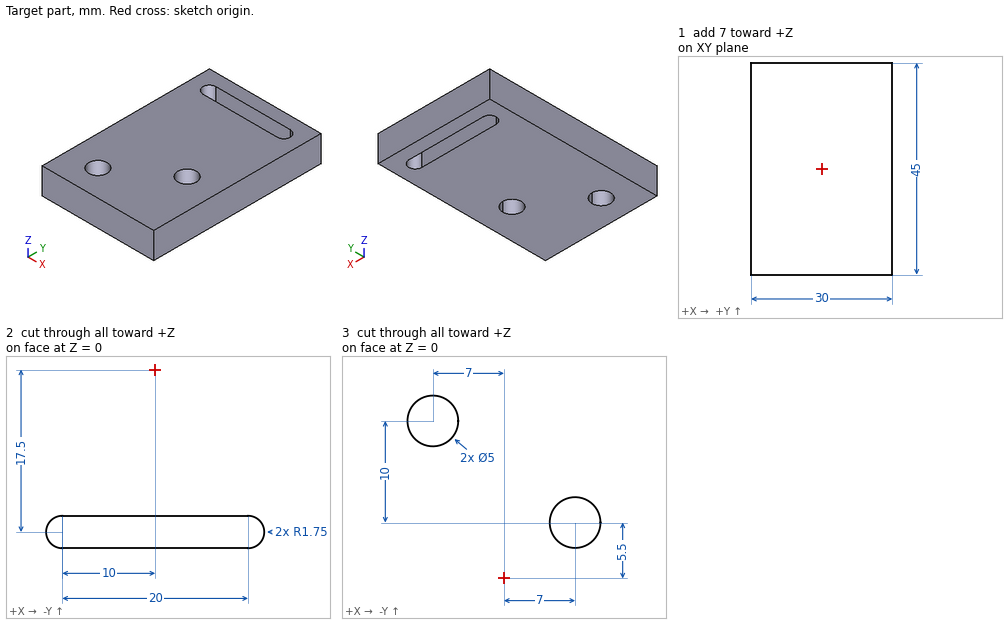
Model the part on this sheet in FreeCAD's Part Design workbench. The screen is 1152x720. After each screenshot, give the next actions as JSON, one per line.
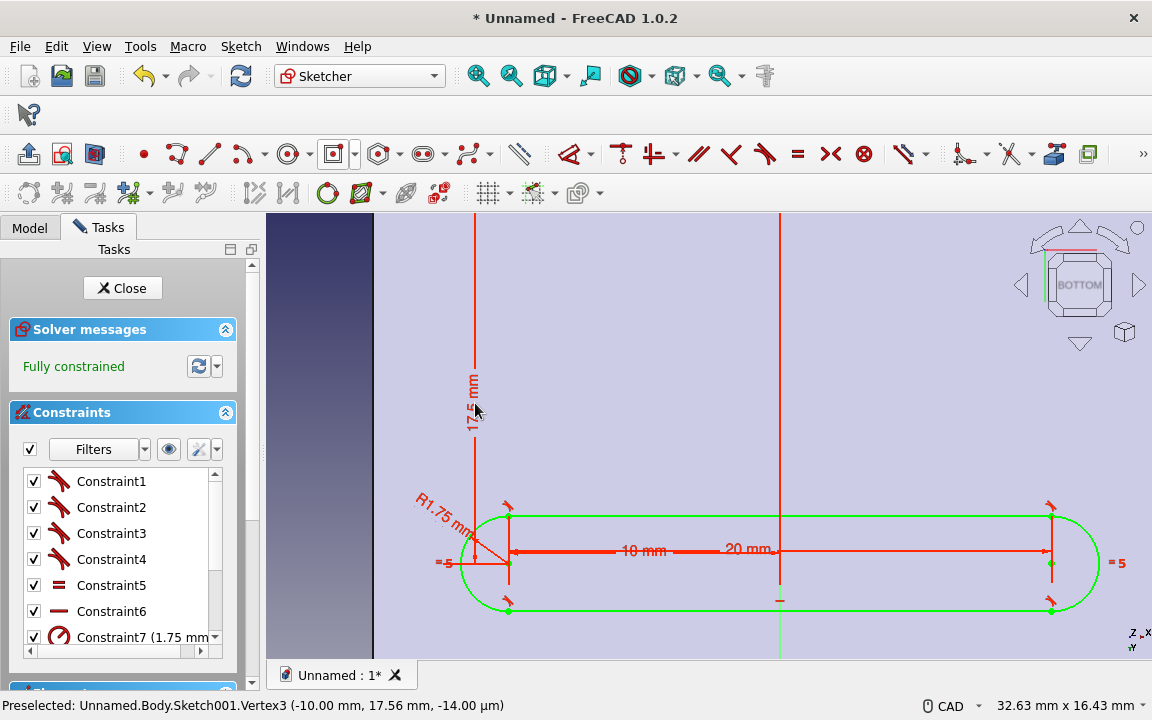
{"action": "left_click", "coordinate": [123, 288]}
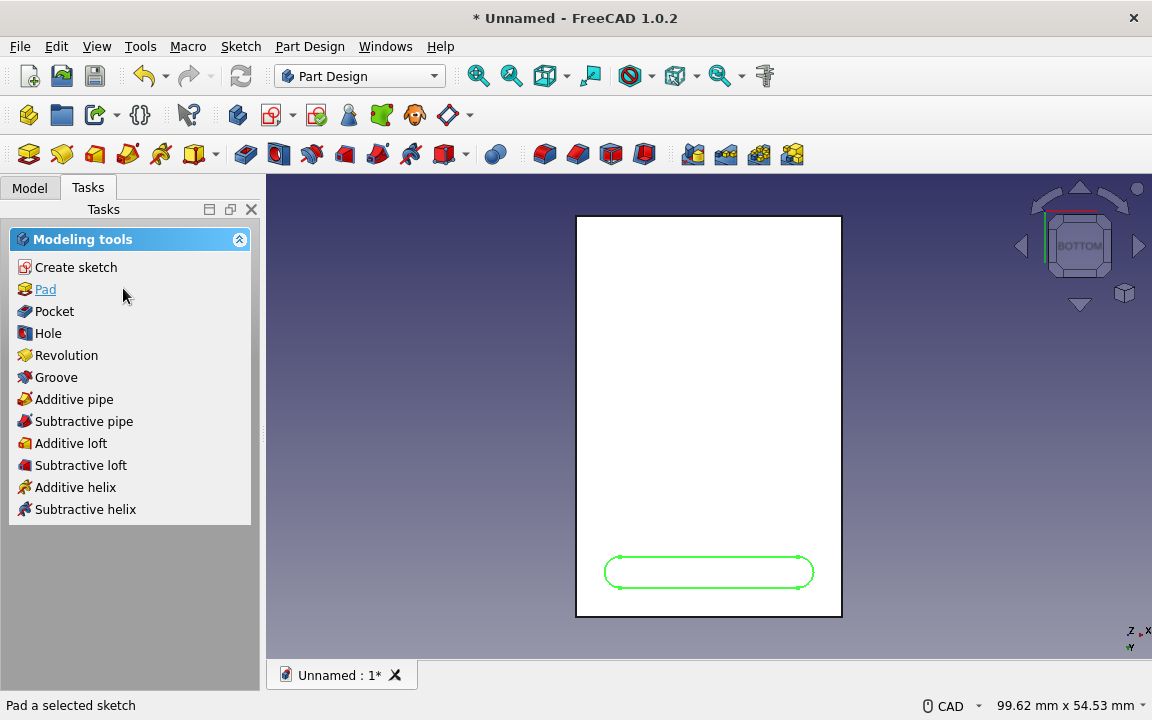
{"action": "left_click", "coordinate": [246, 154]}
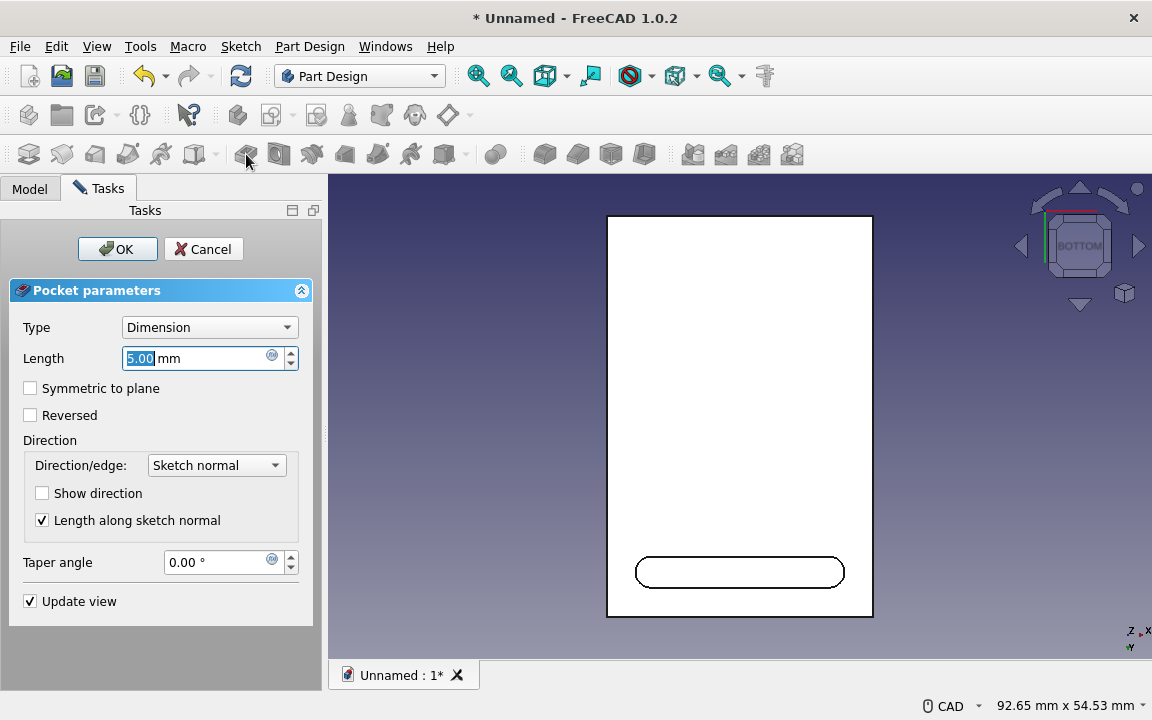
{"action": "left_click", "coordinate": [210, 328]}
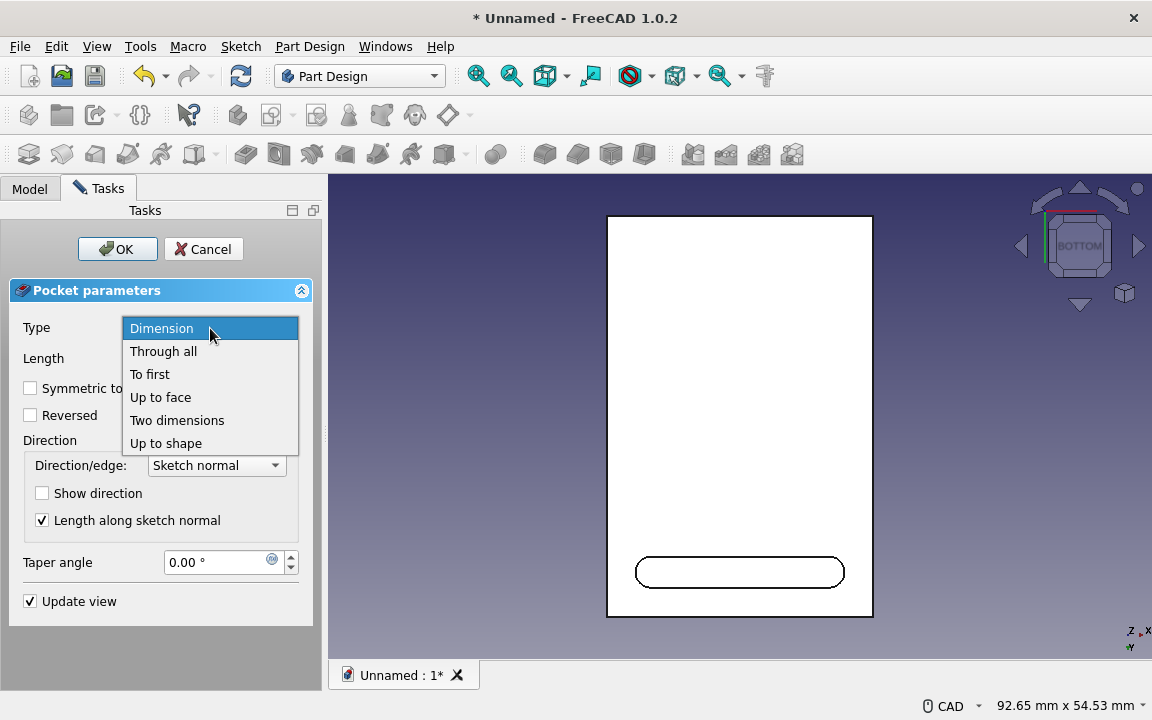
{"action": "left_click", "coordinate": [208, 352]}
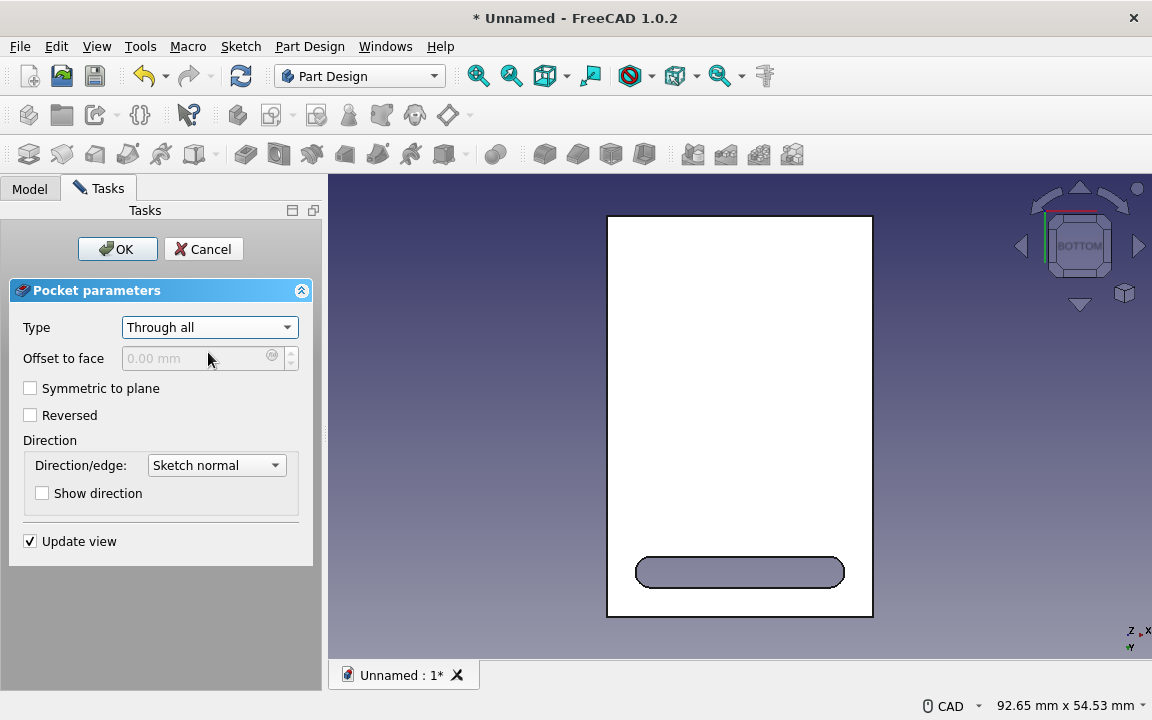
{"action": "left_click", "coordinate": [118, 249]}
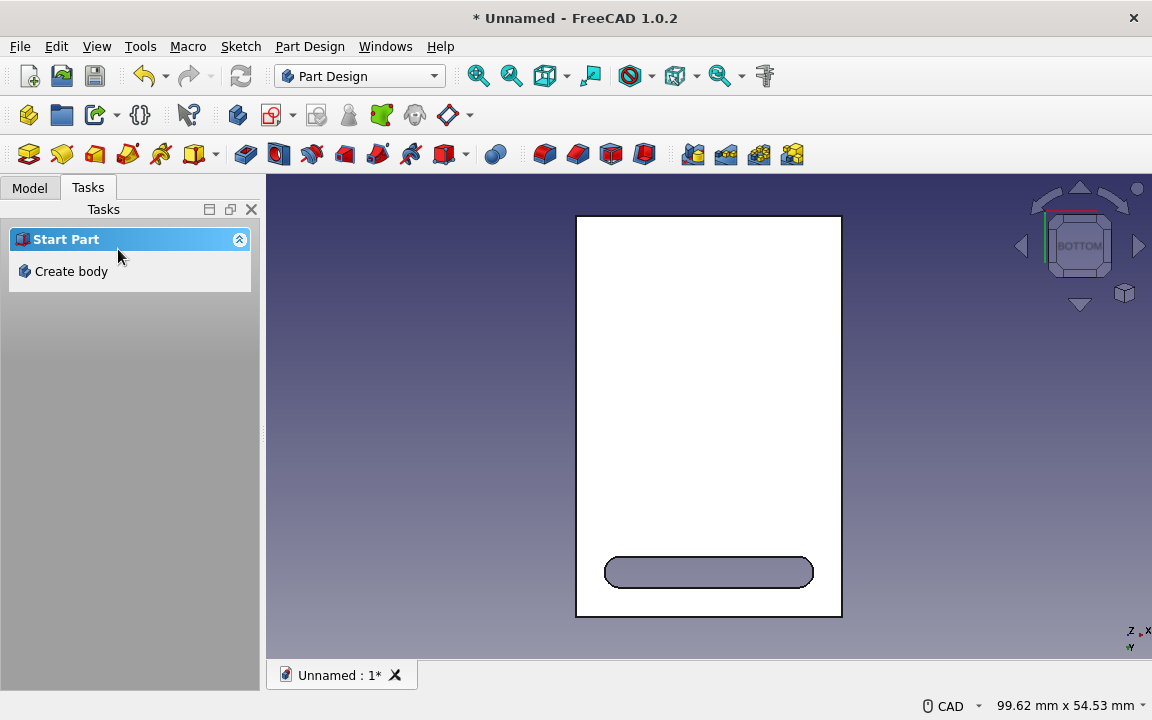
{"action": "left_click", "coordinate": [709, 416]}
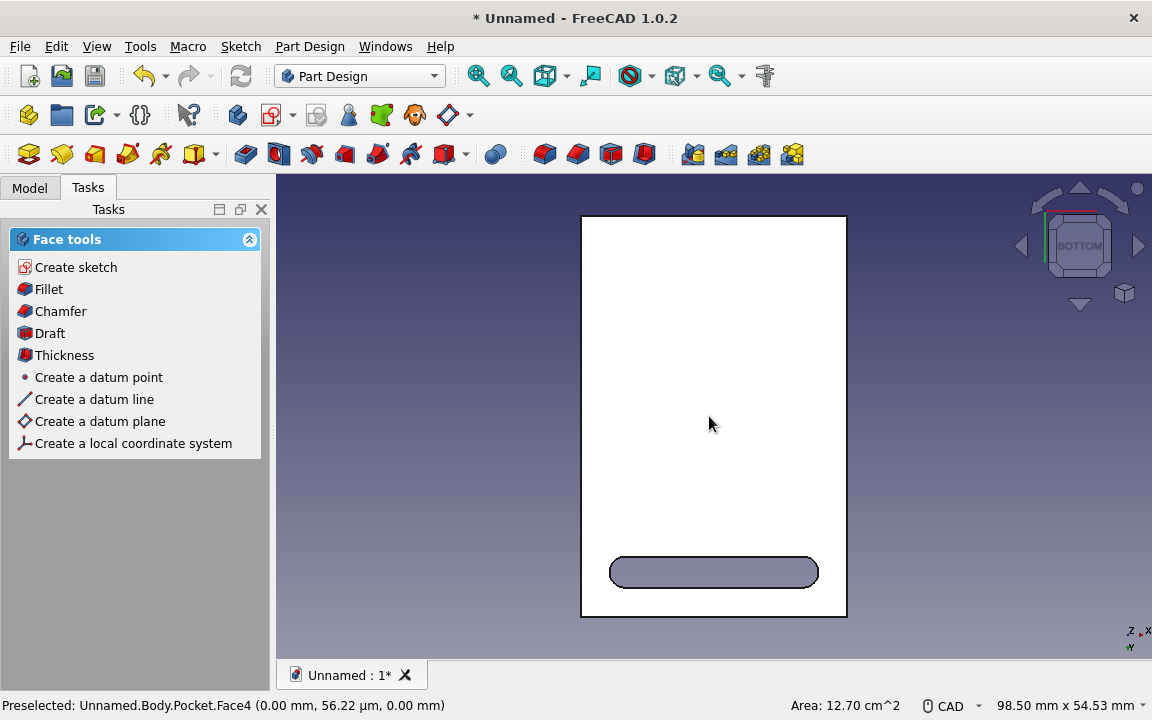
{"action": "left_click", "coordinate": [270, 116]}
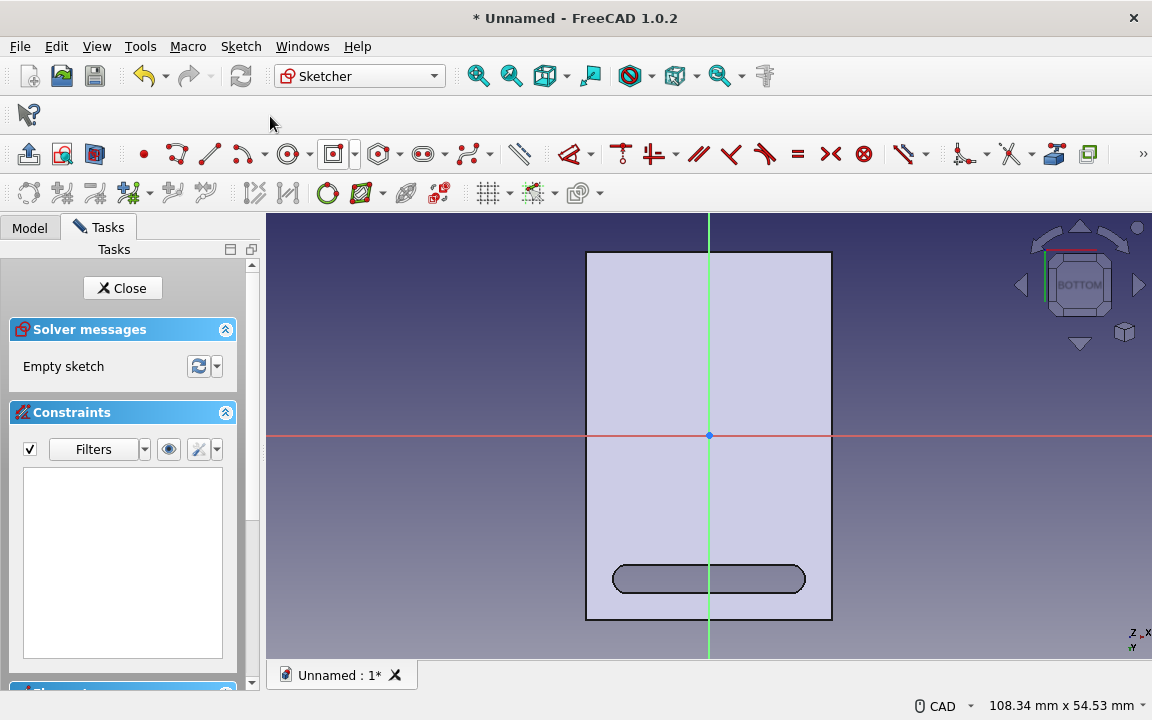
{"action": "scroll", "coordinate": [792, 273], "scroll_direction": "up", "scroll_amount": 3}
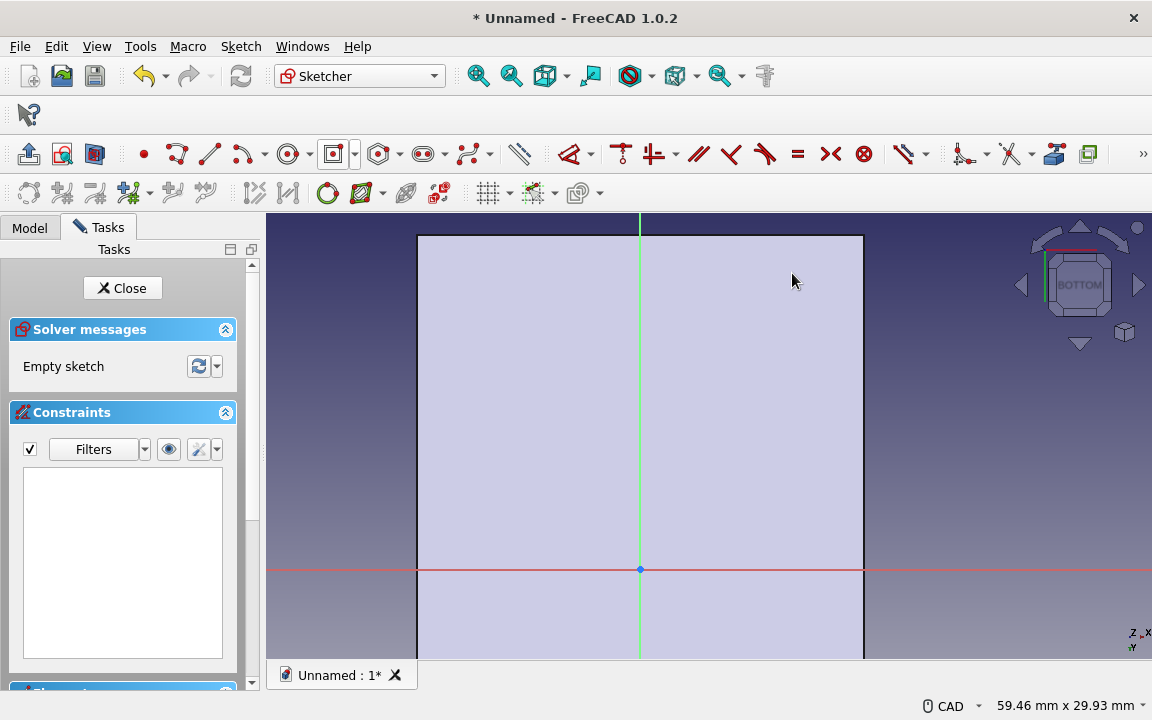
{"action": "left_click", "coordinate": [288, 154]}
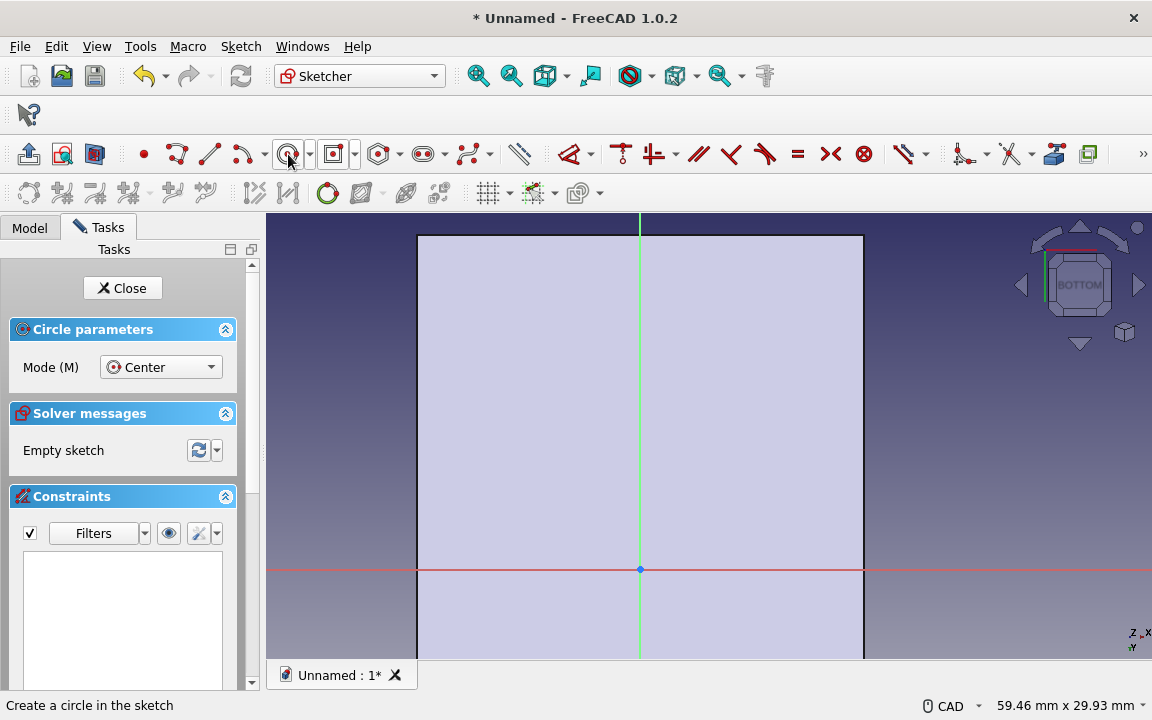
{"action": "left_click", "coordinate": [536, 339]}
{"action": "left_click", "coordinate": [562, 313]}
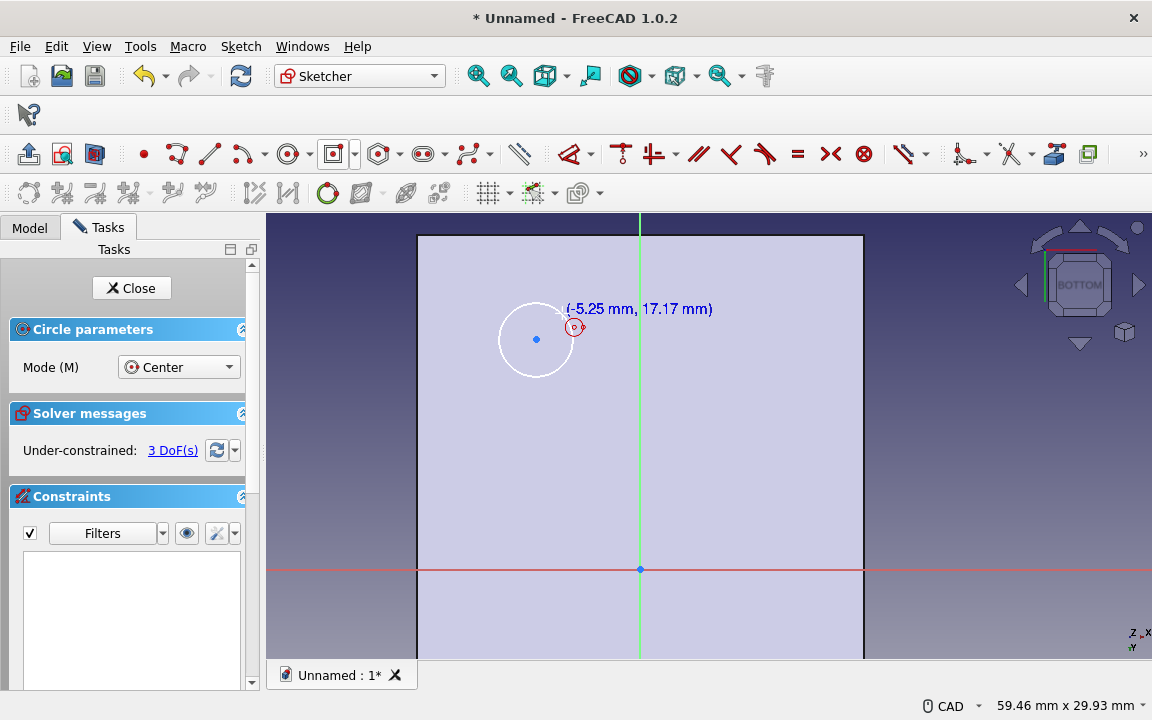
{"action": "left_click", "coordinate": [745, 488]}
{"action": "left_click", "coordinate": [771, 462]}
{"action": "key", "text": "Escape"}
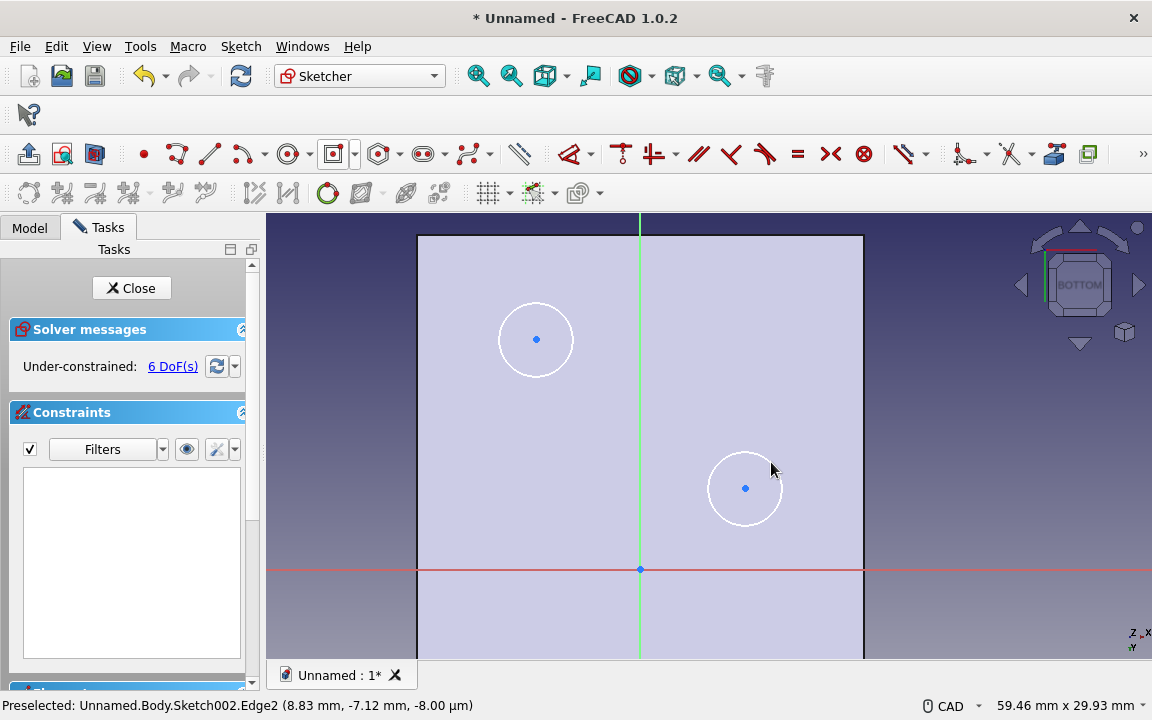
{"action": "left_click", "coordinate": [562, 314]}